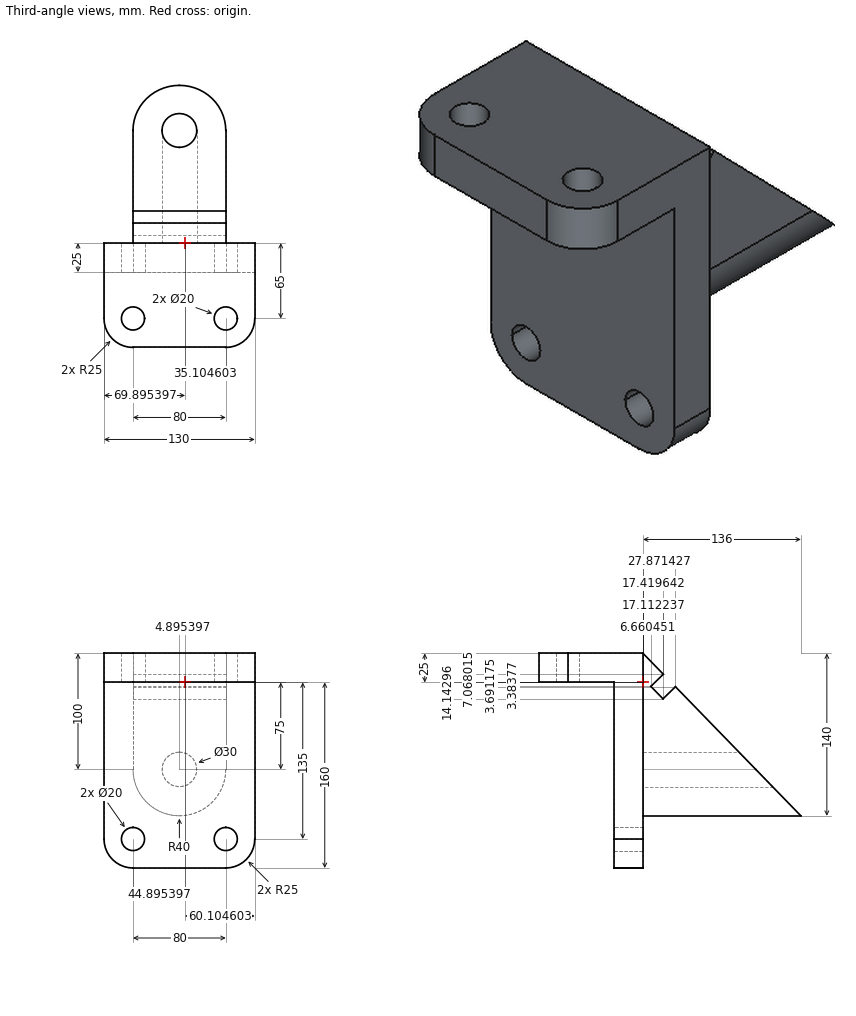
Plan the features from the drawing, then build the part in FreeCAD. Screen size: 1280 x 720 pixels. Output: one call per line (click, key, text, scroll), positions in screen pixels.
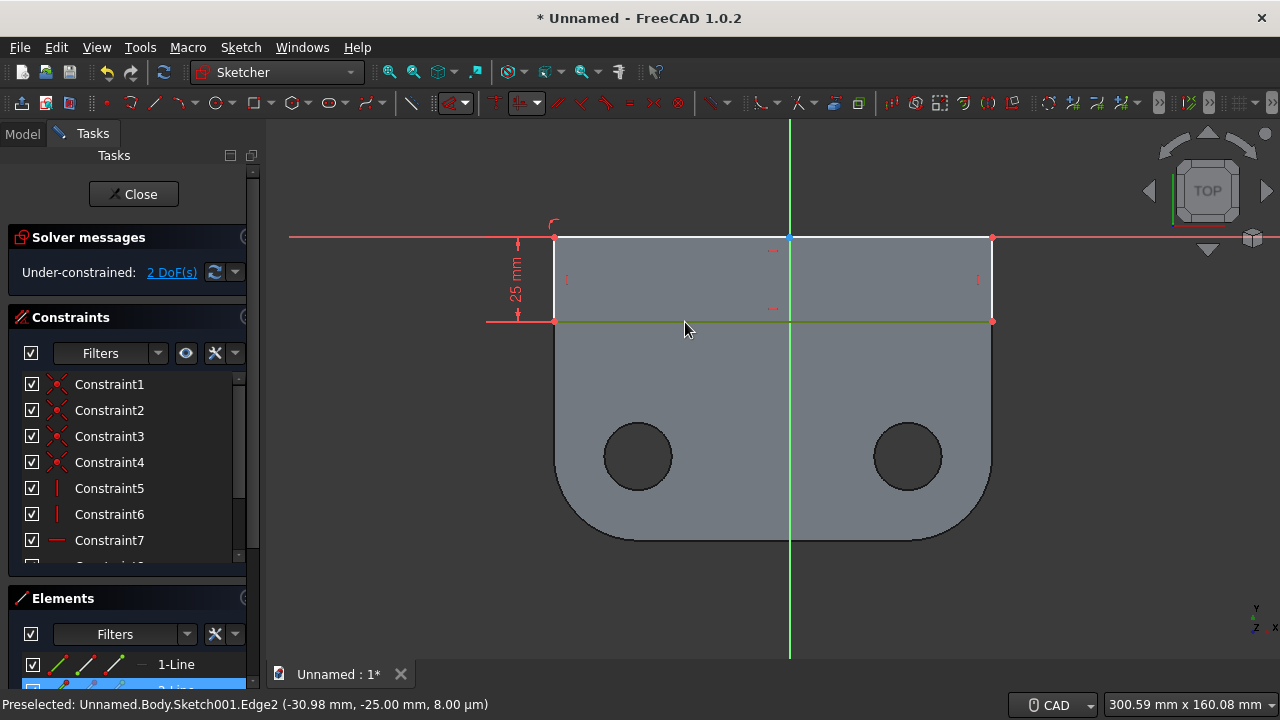
key(l)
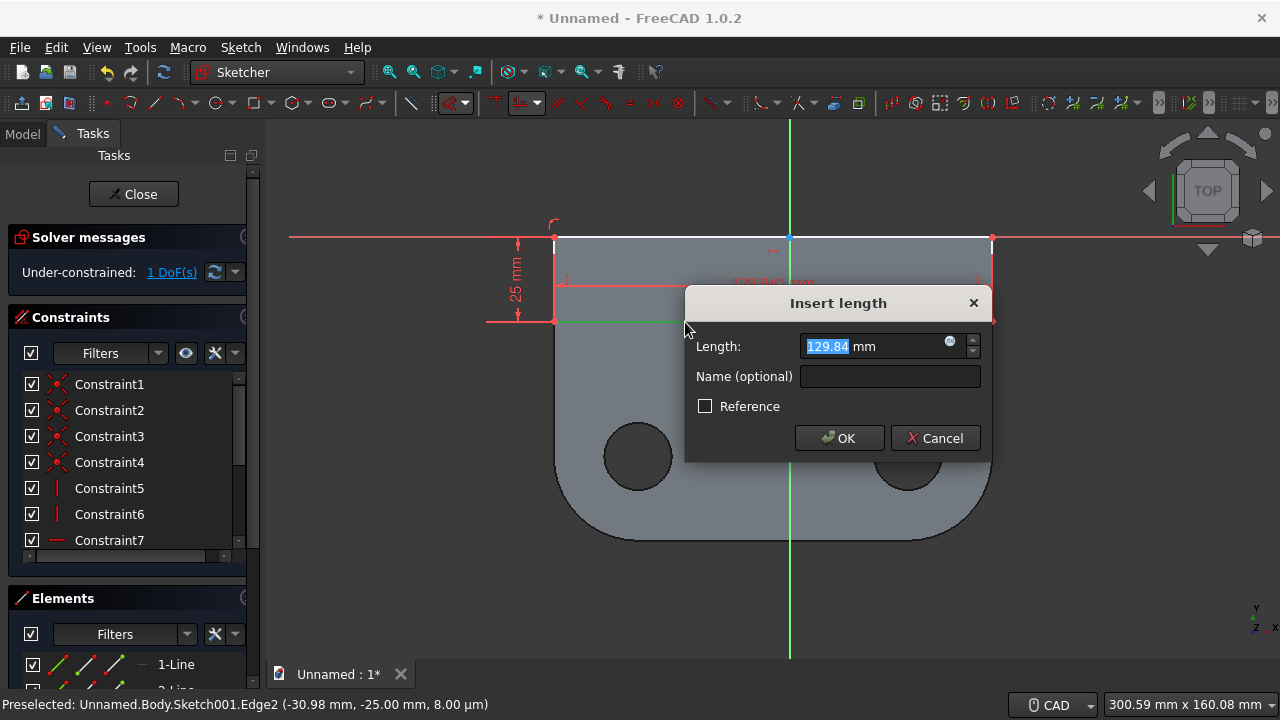
text(130)
key(Return)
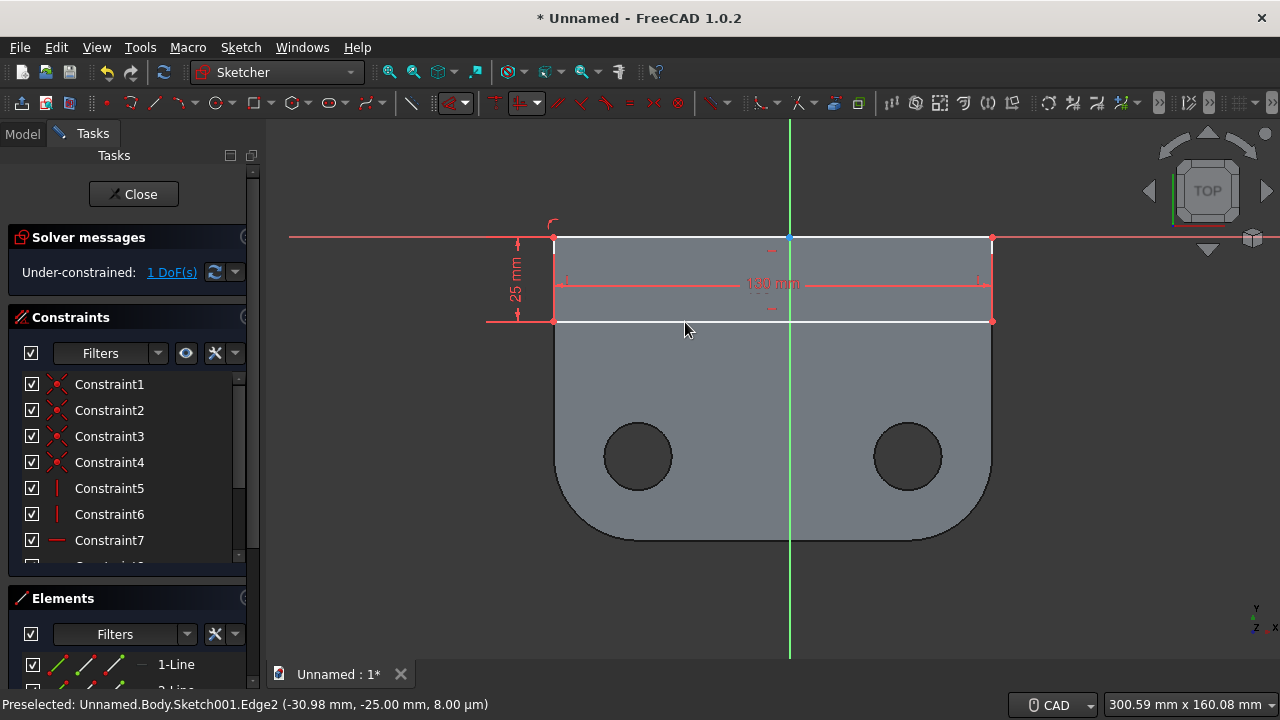
click(554, 237)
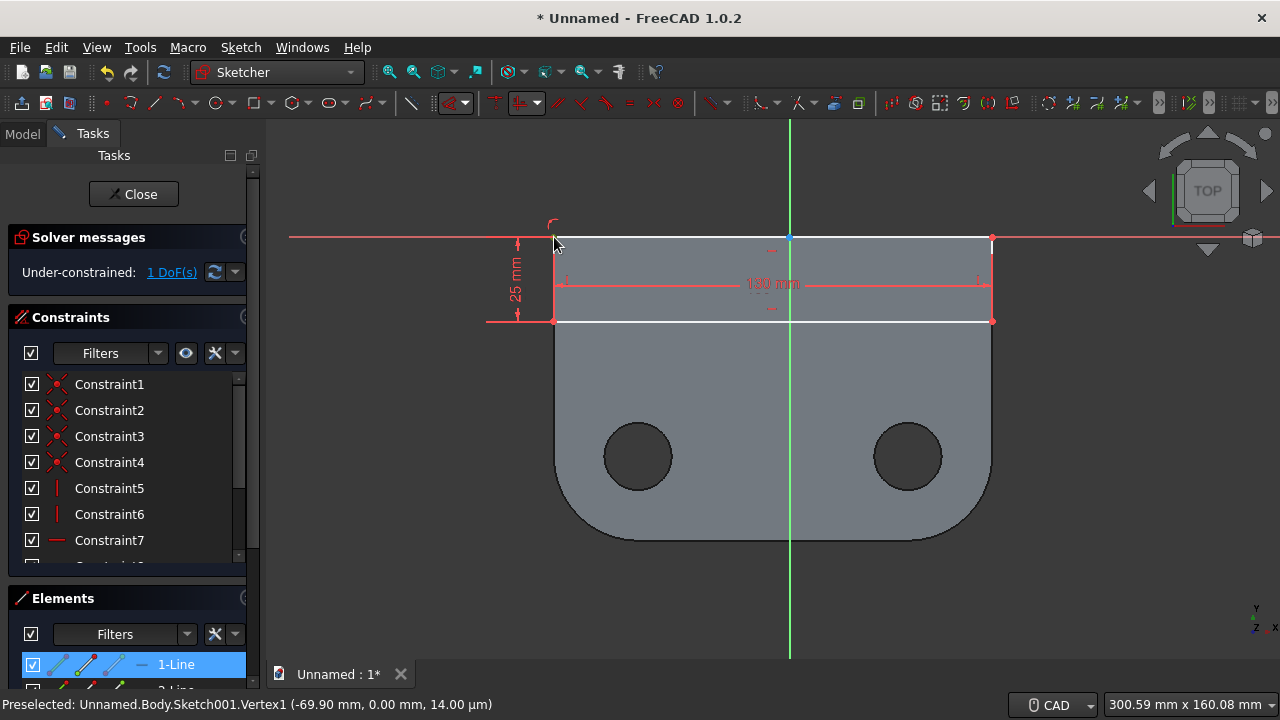
click(468, 104)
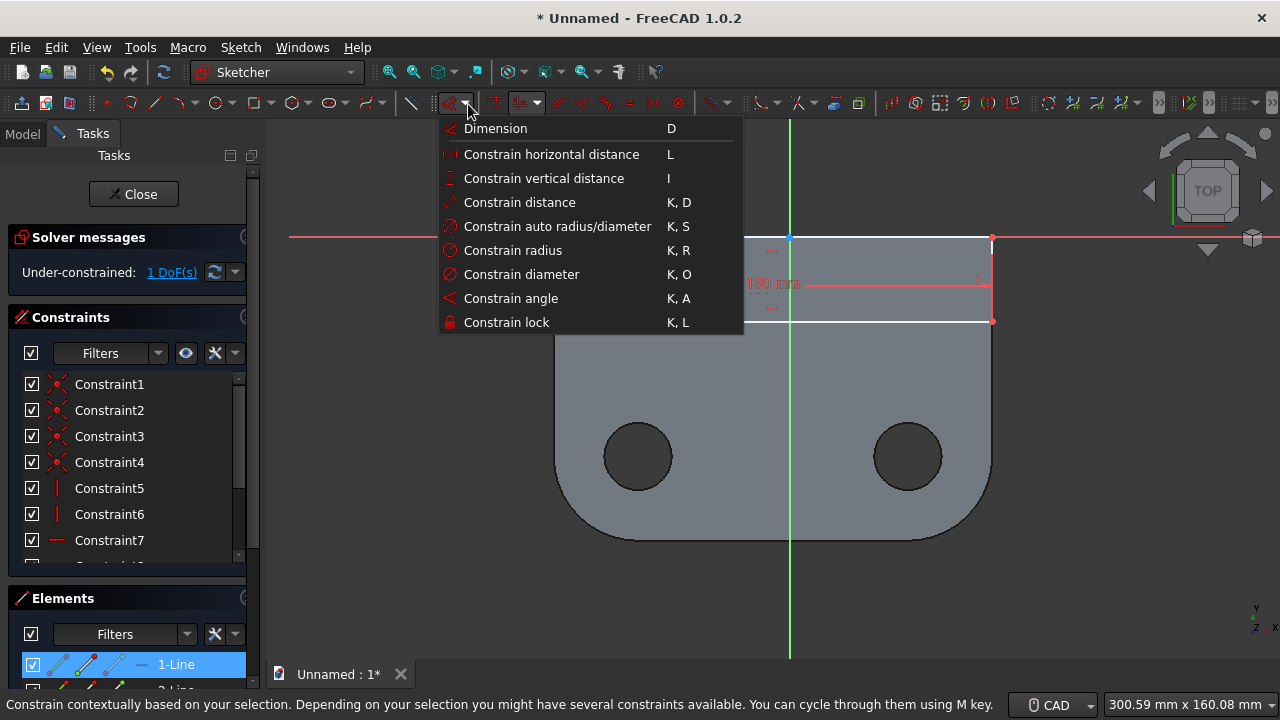
click(591, 154)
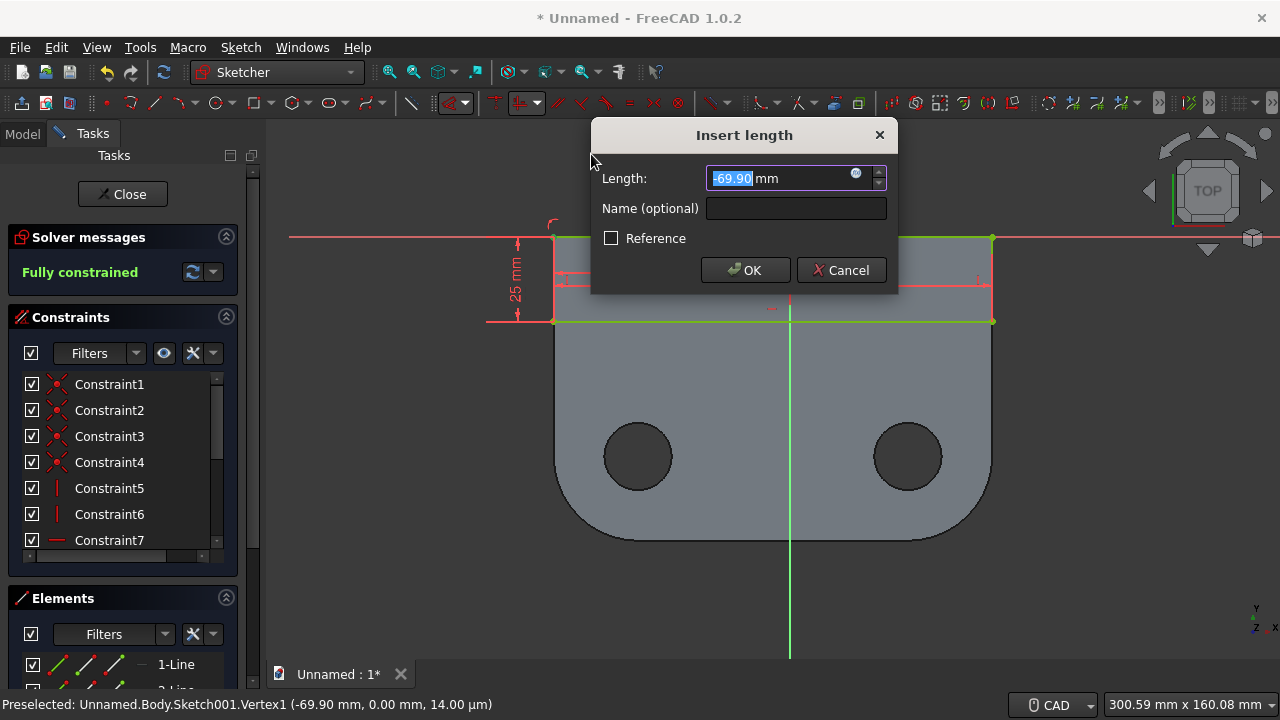
text(-69.895397)
key(Return)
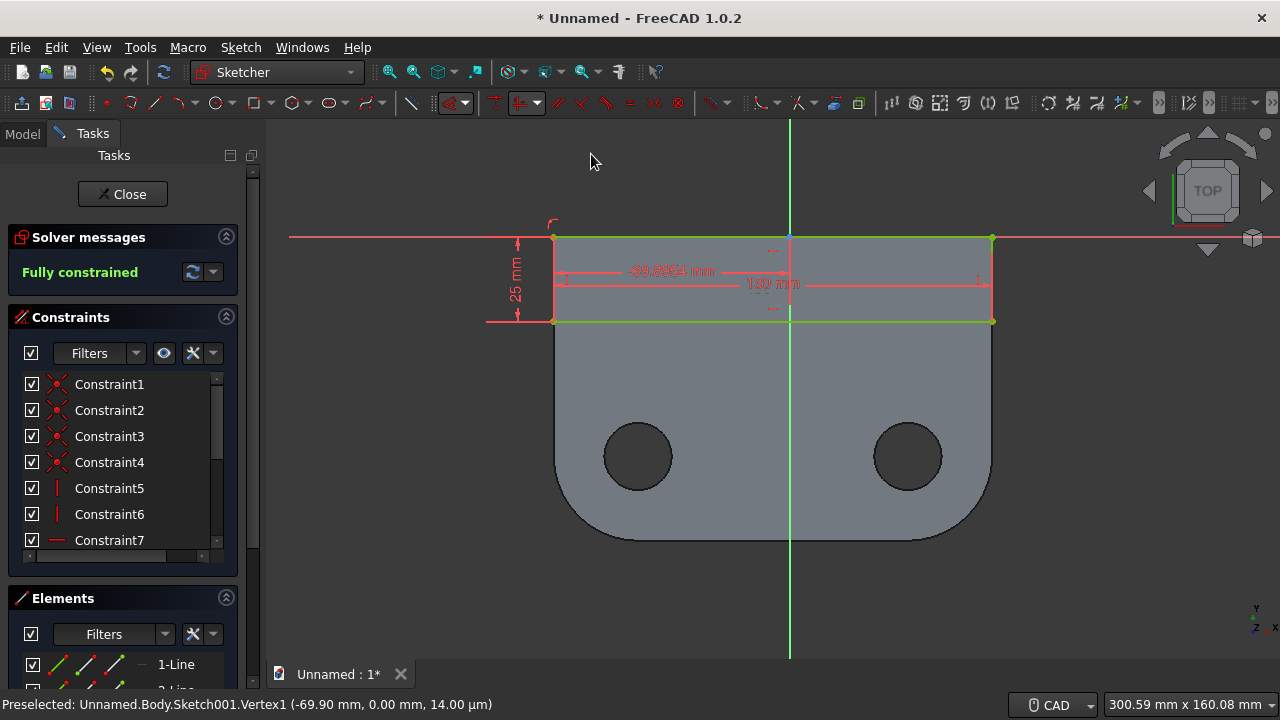
click(123, 194)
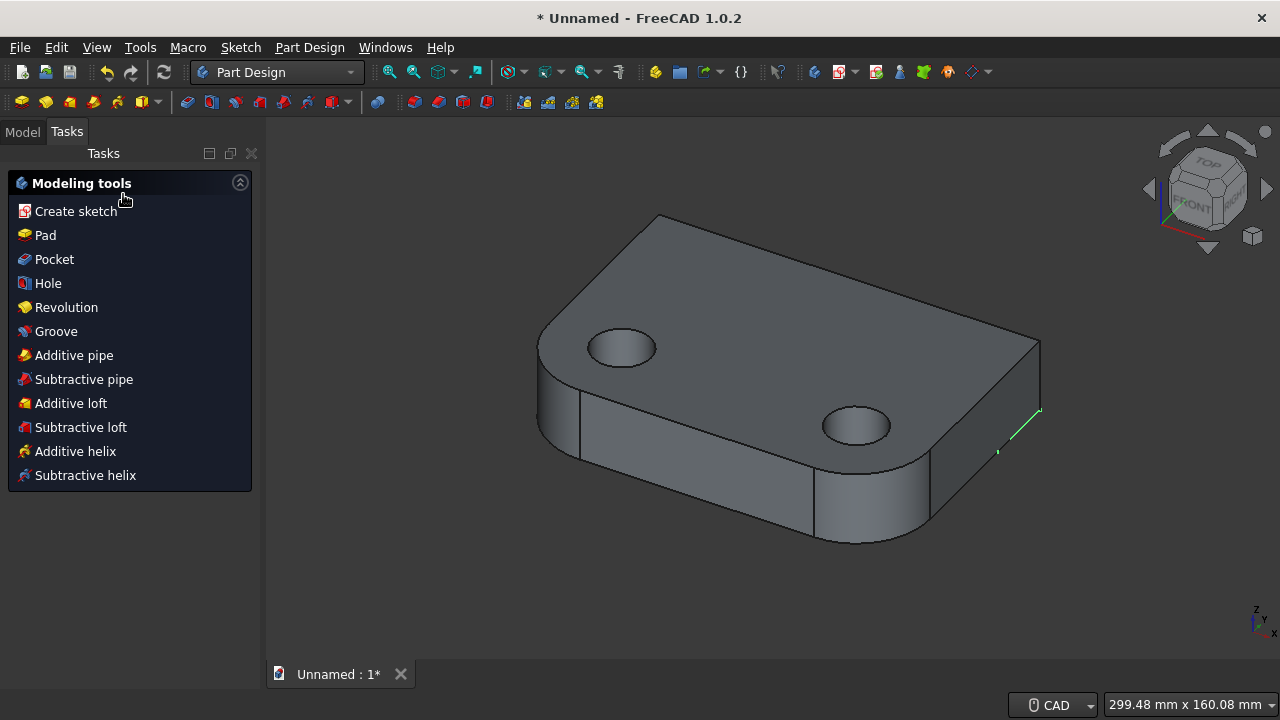
click(22, 102)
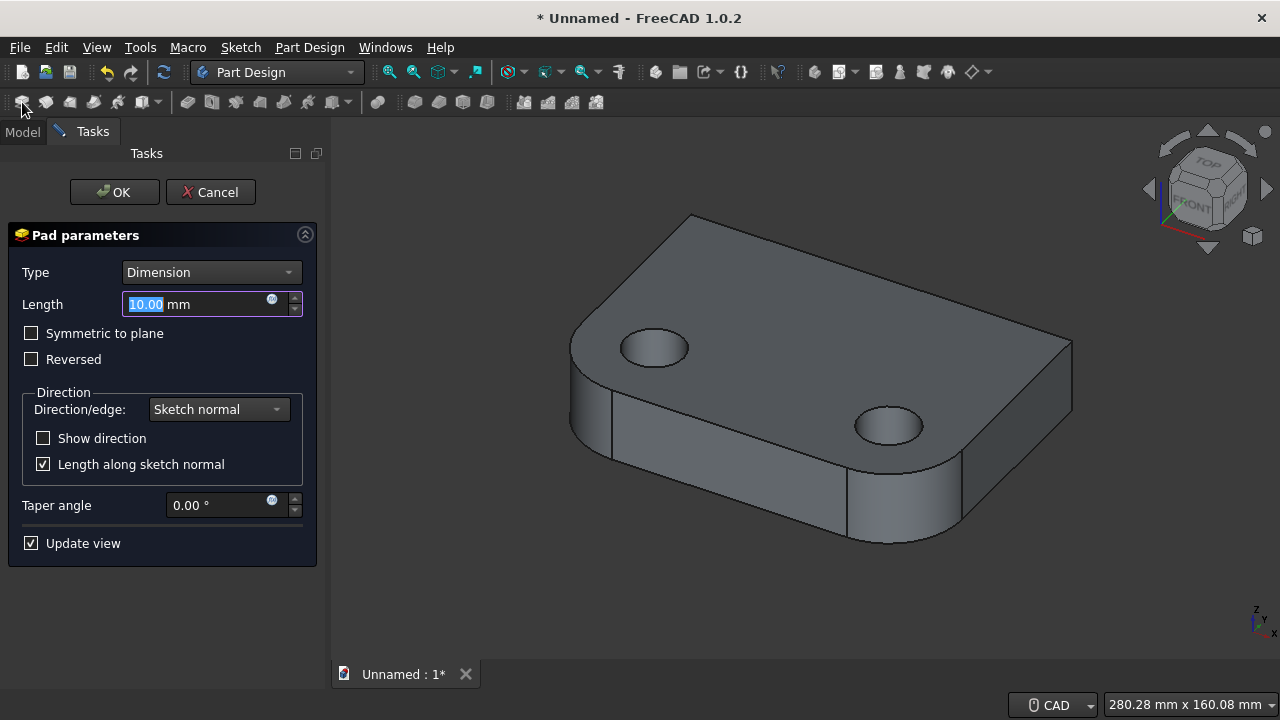
text(160)
key(Tab)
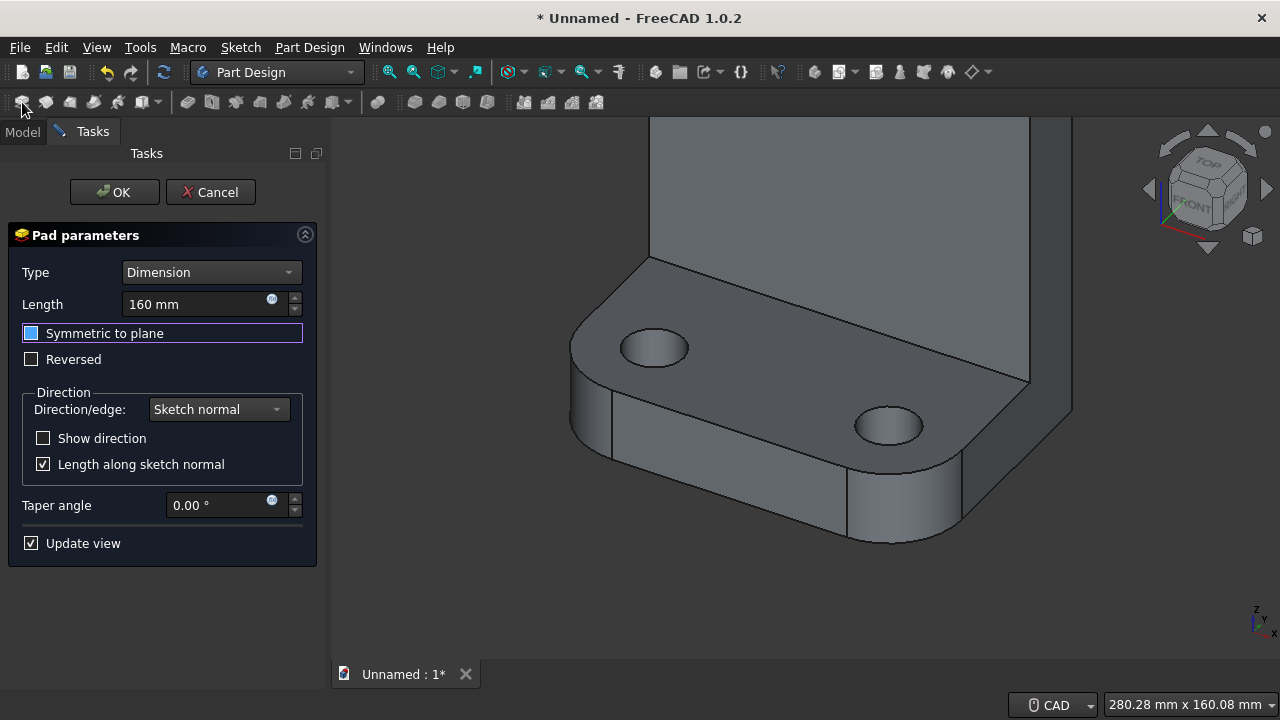
click(30, 359)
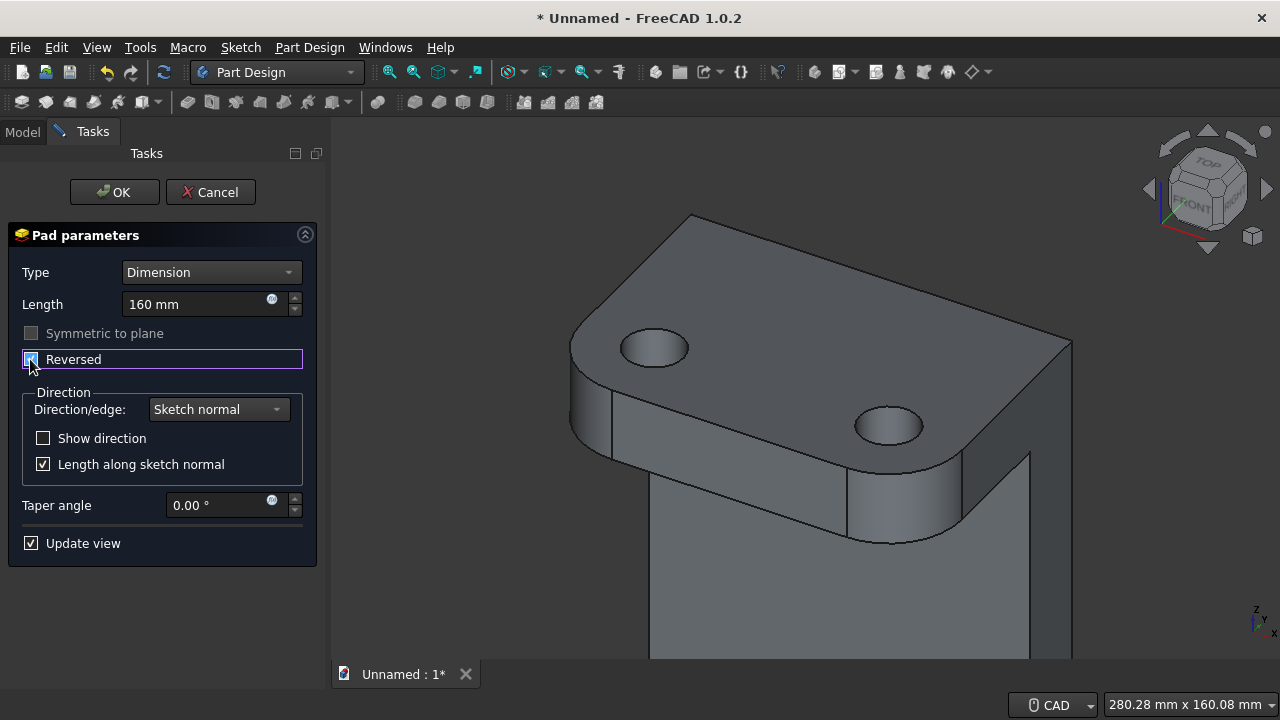
click(115, 192)